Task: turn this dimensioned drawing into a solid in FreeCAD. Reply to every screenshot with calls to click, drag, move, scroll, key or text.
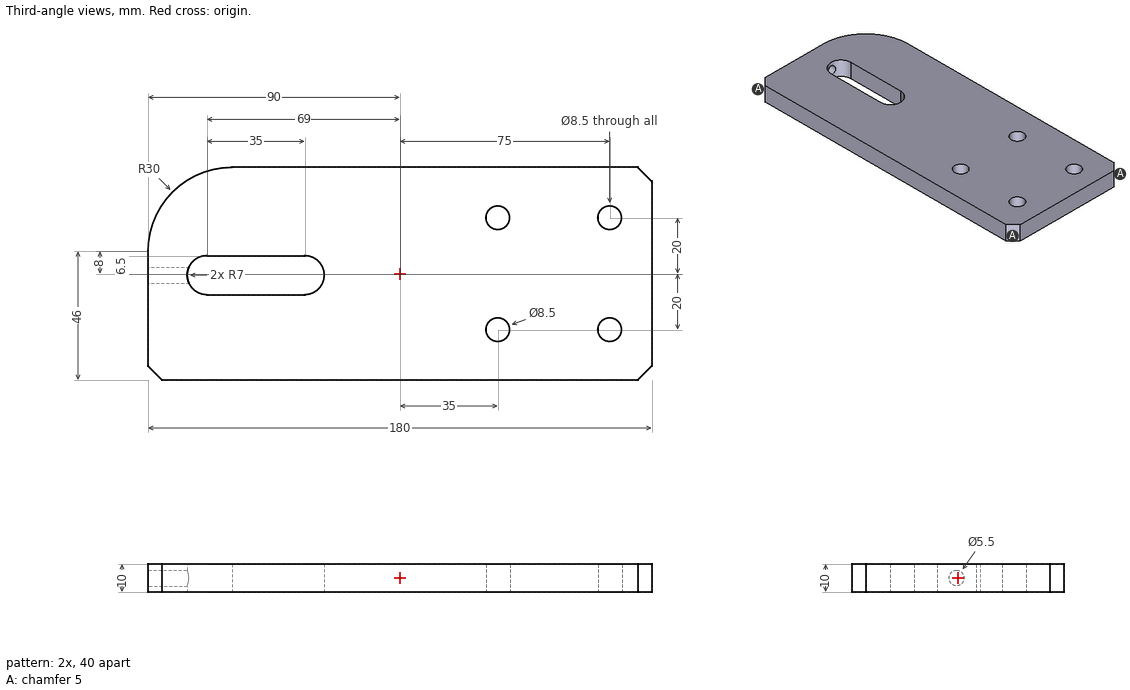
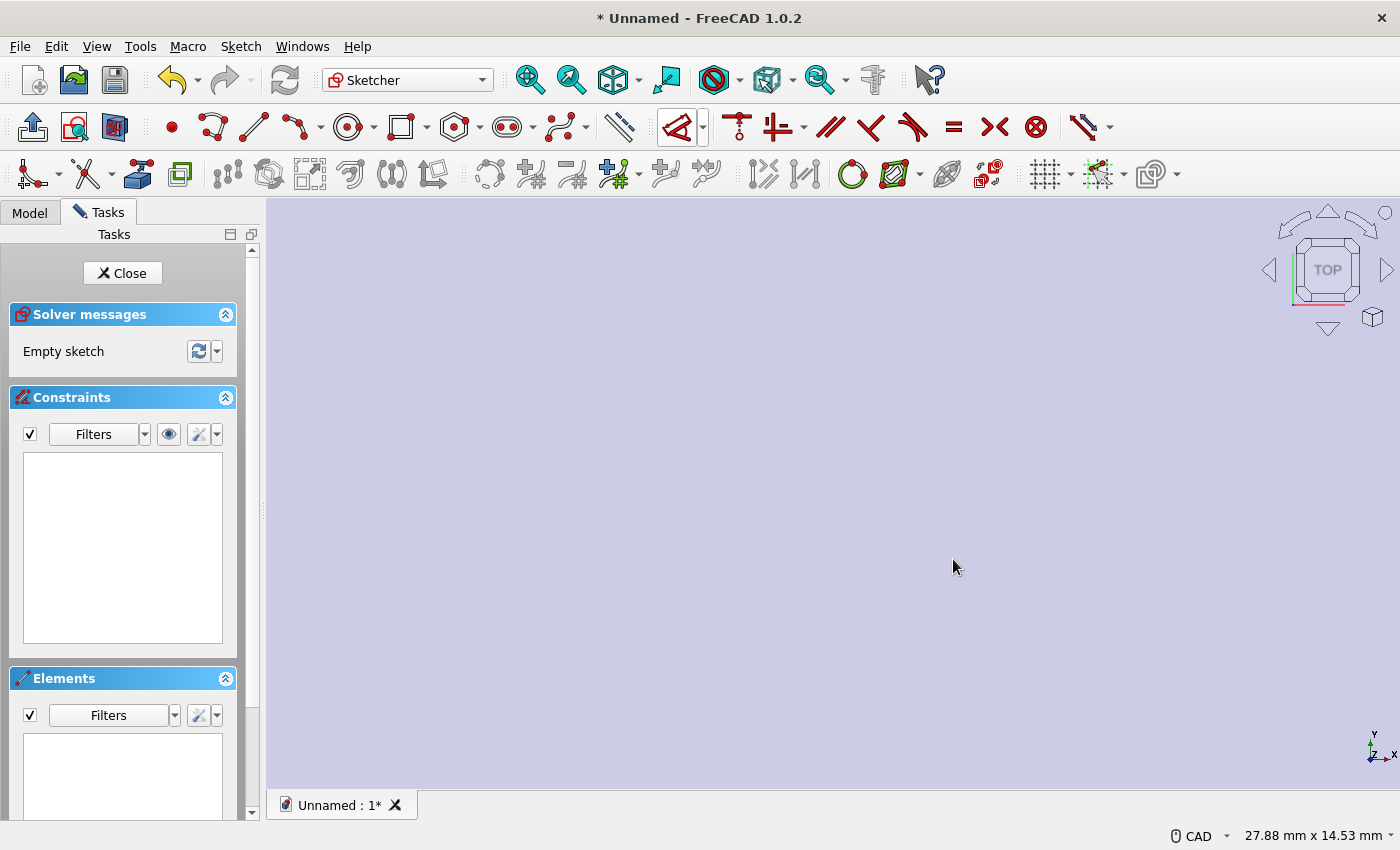
key(g)
key(c)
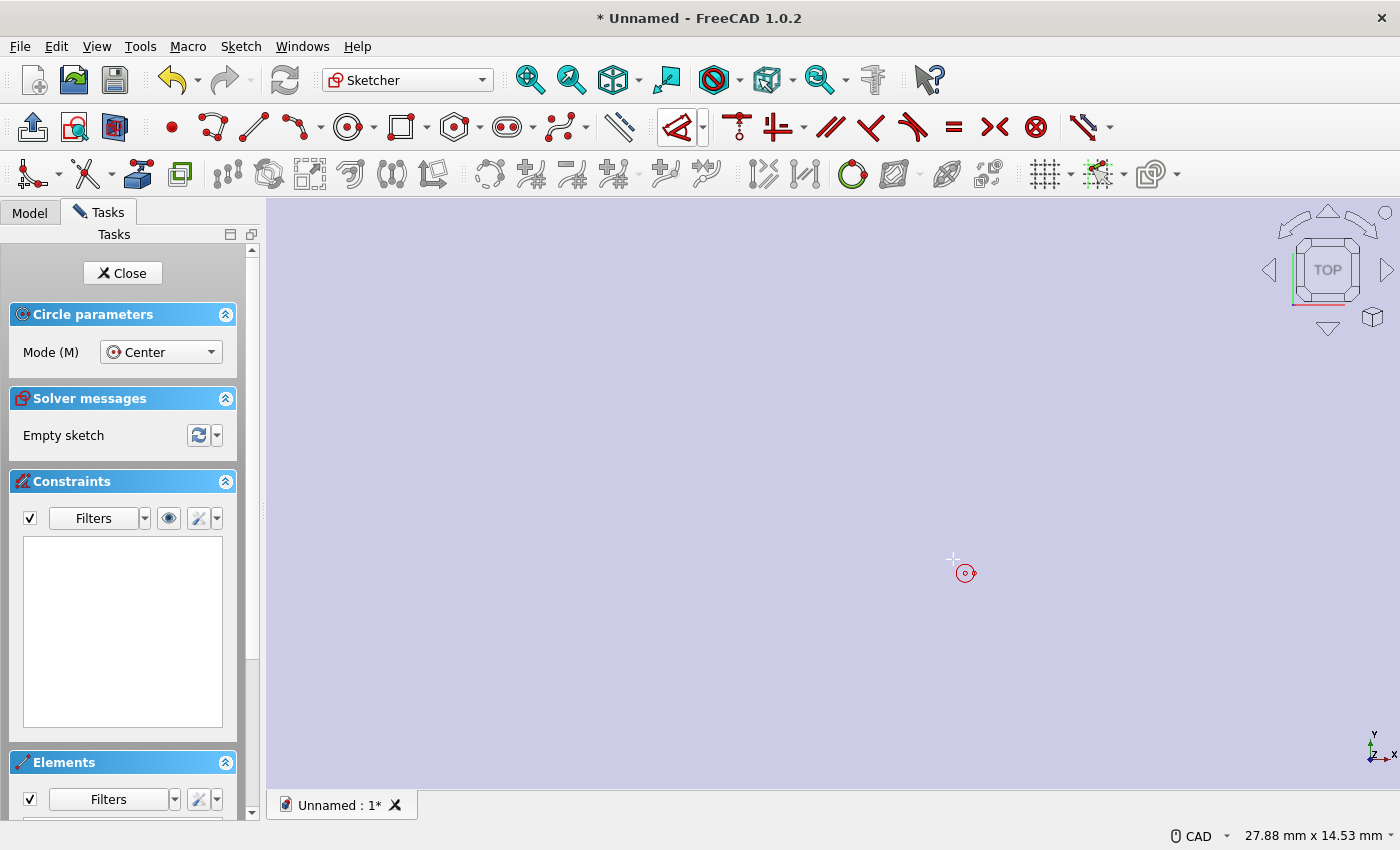
click(753, 483)
click(876, 361)
key(Escape)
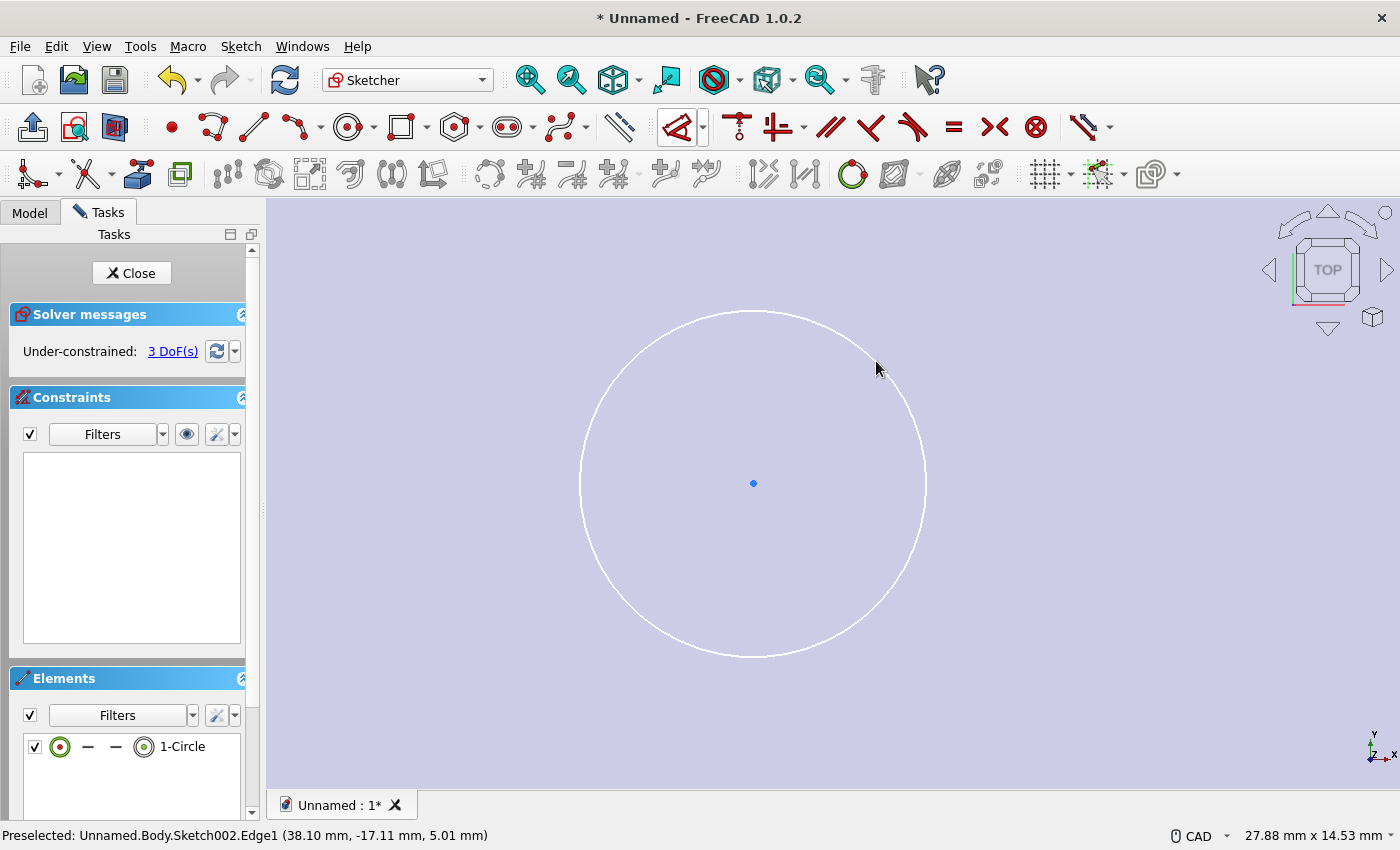
click(875, 361)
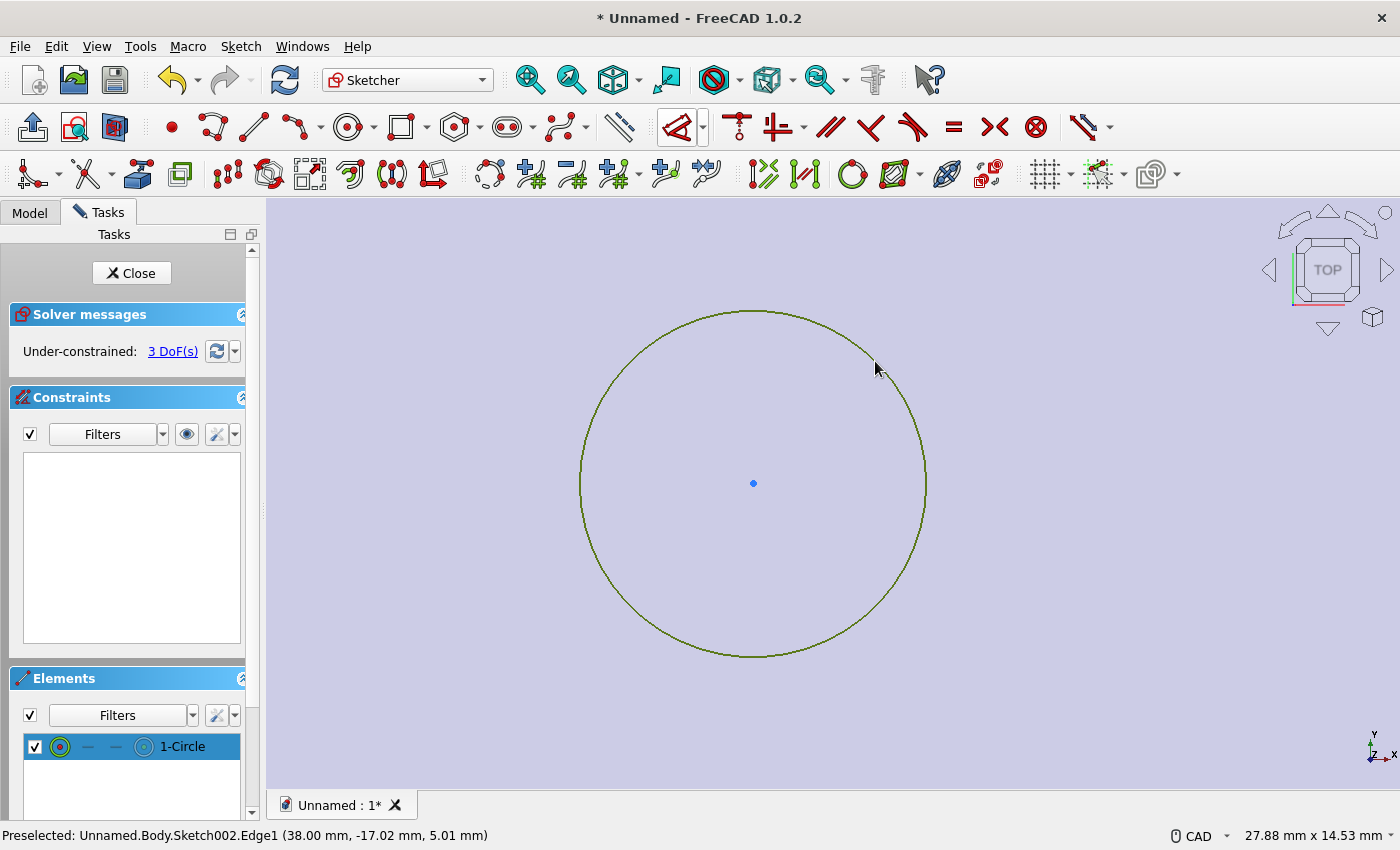
click(702, 128)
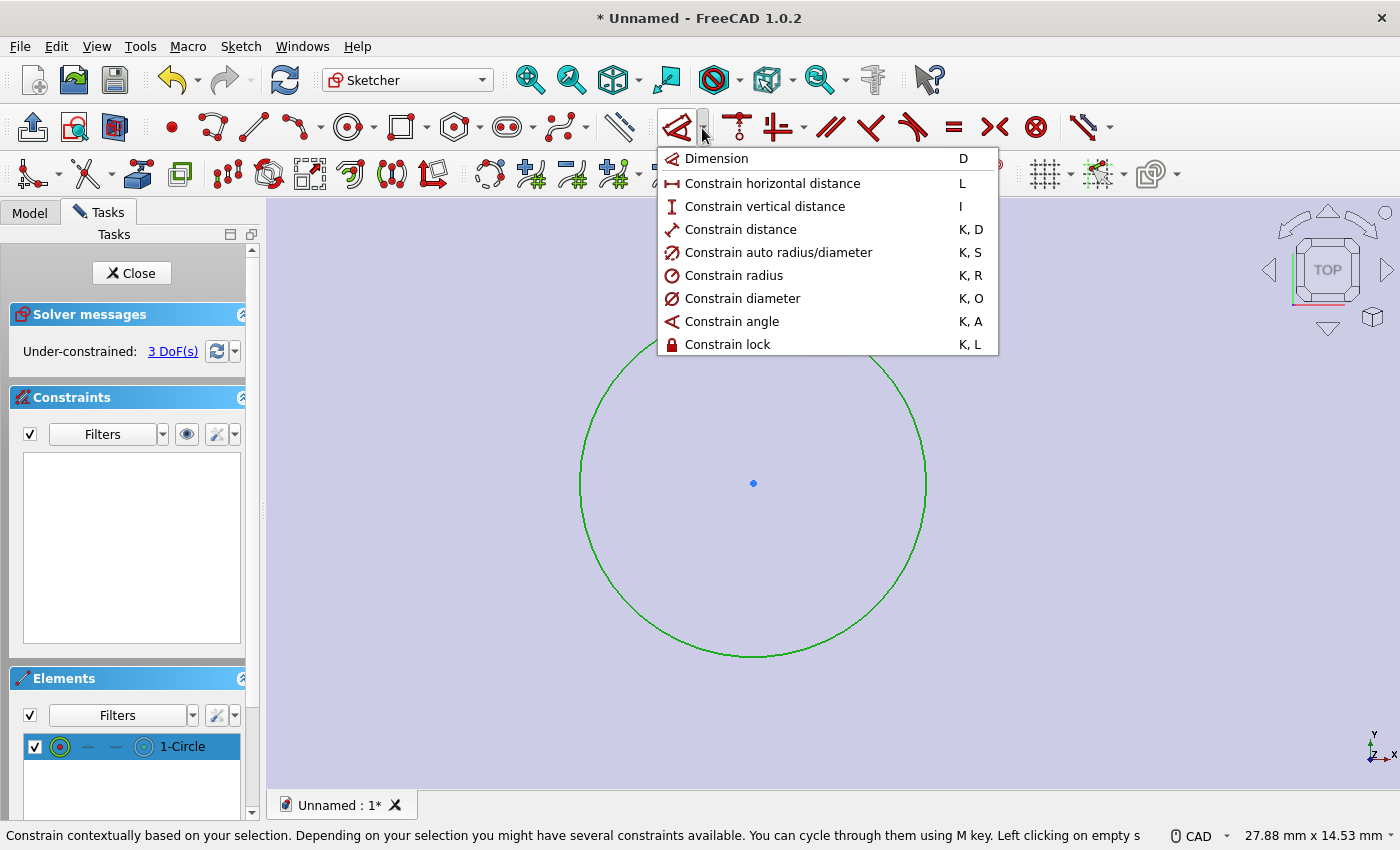
click(828, 298)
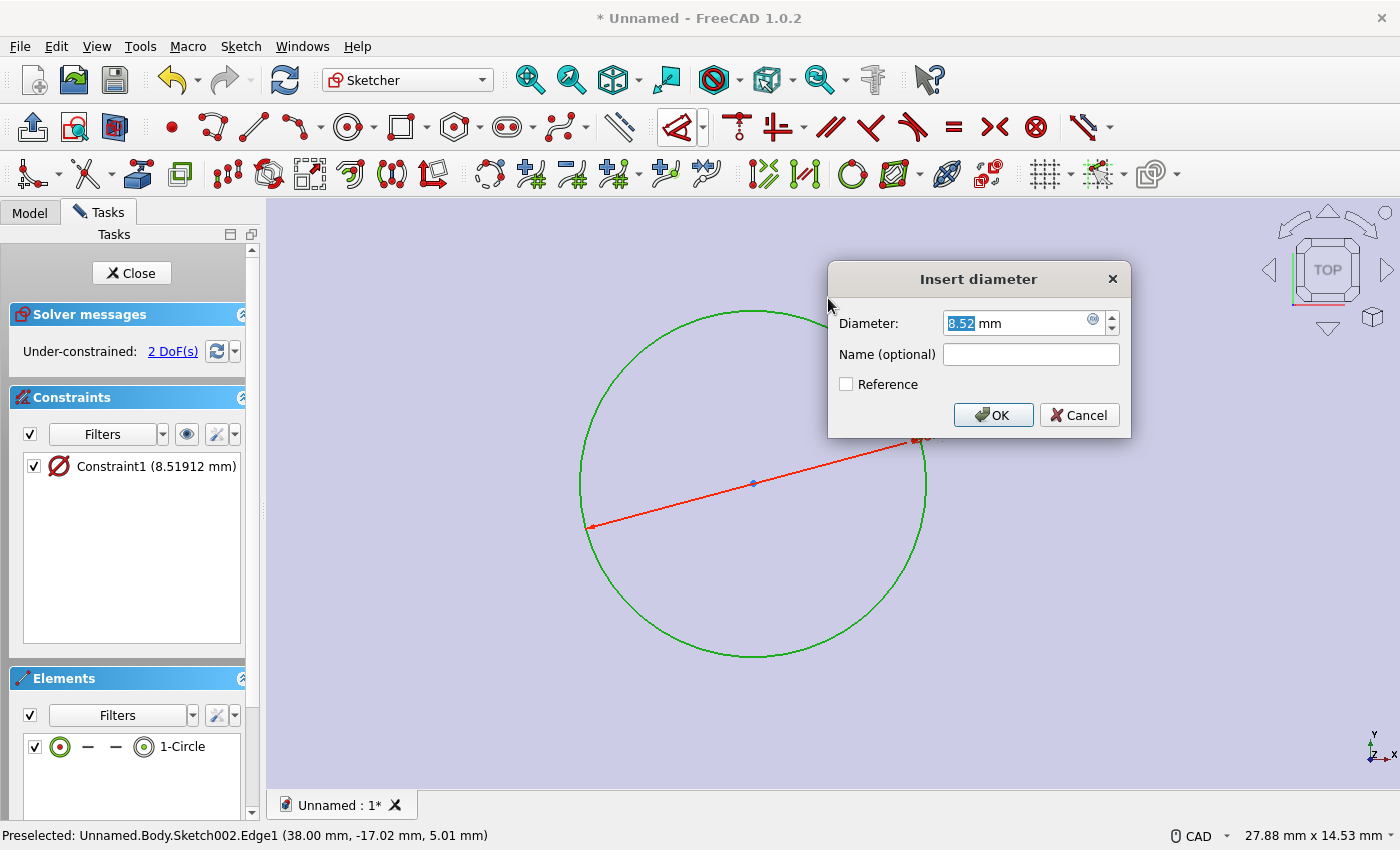
text(8.5)
key(Return)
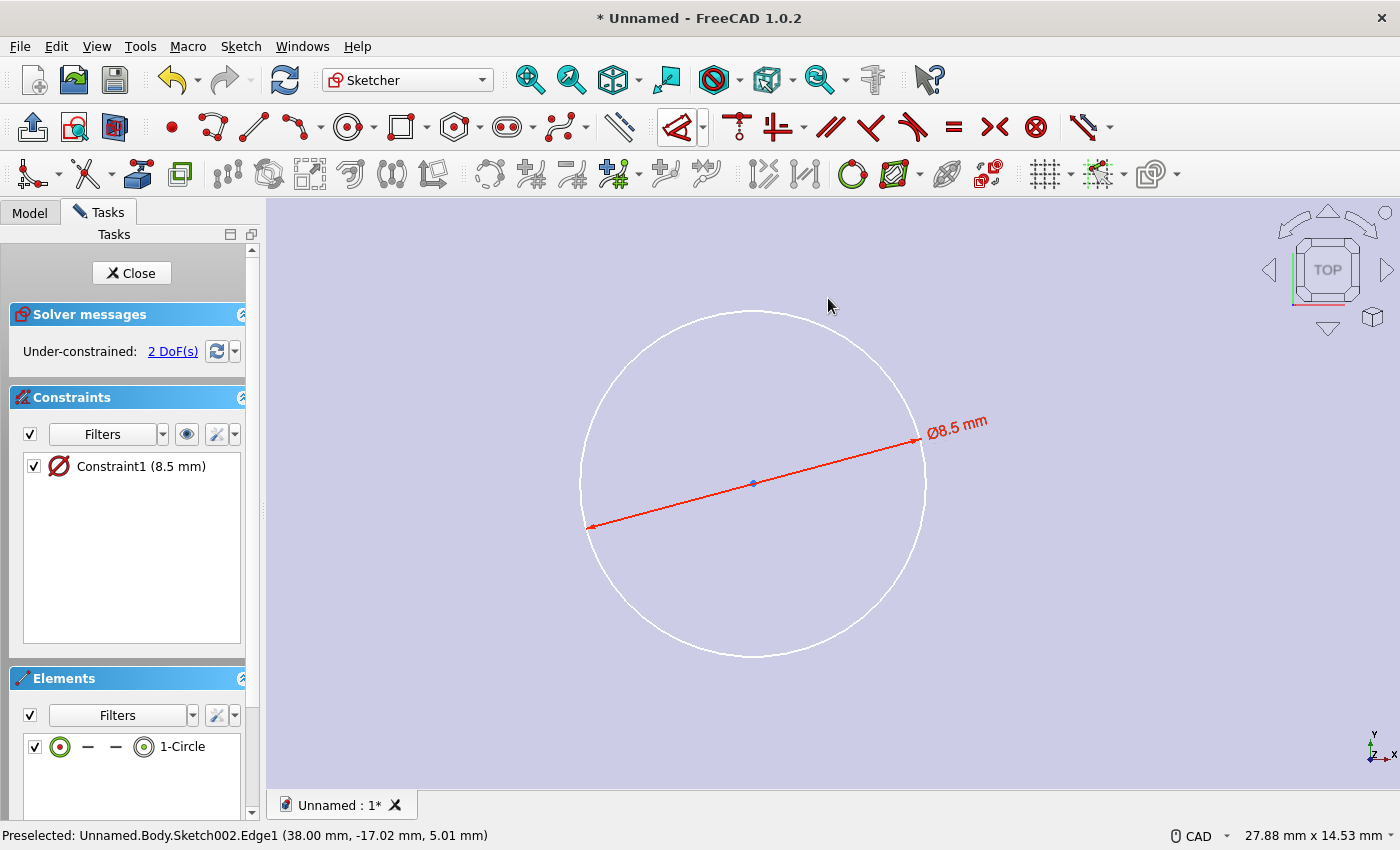
click(753, 484)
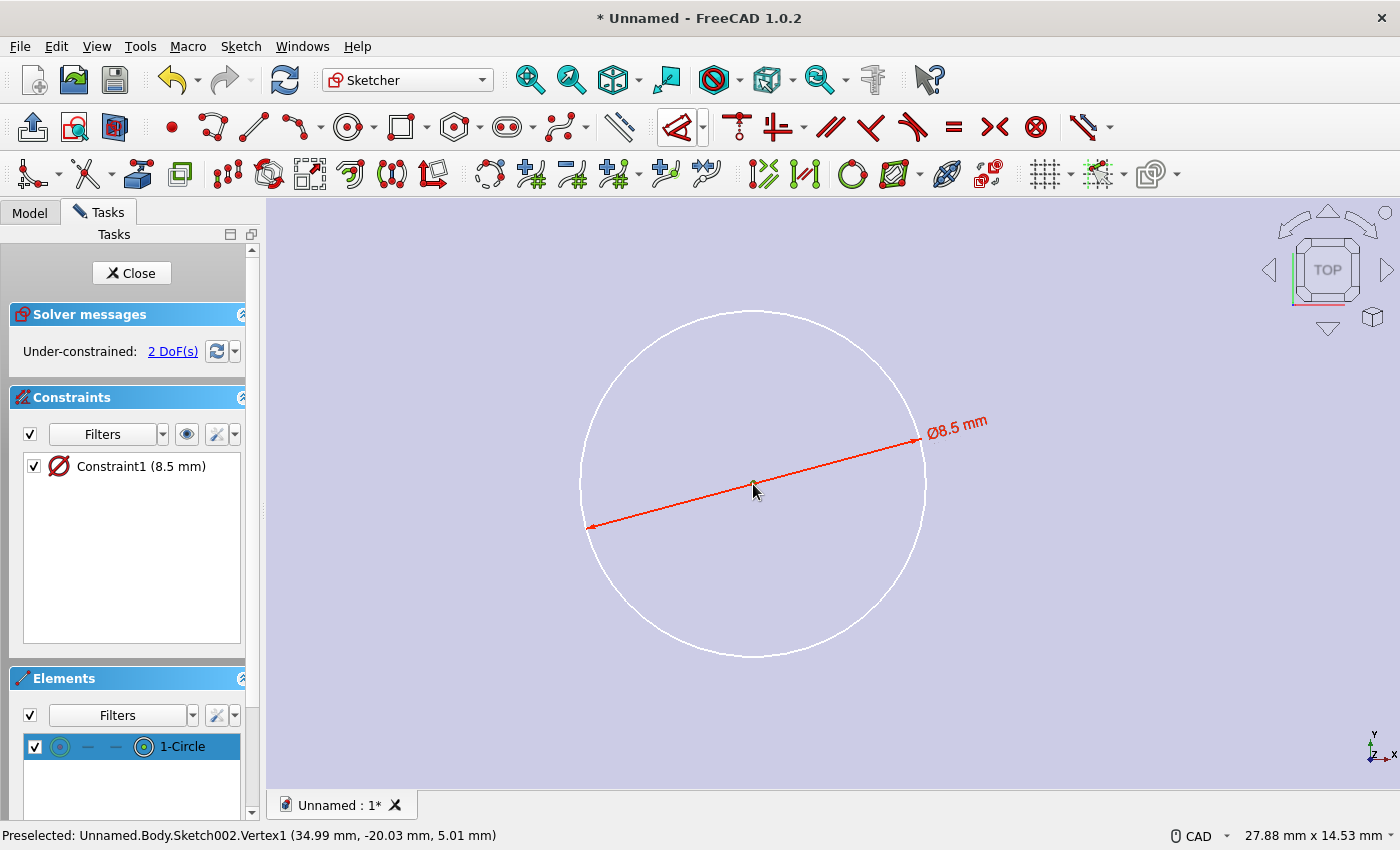
key(l)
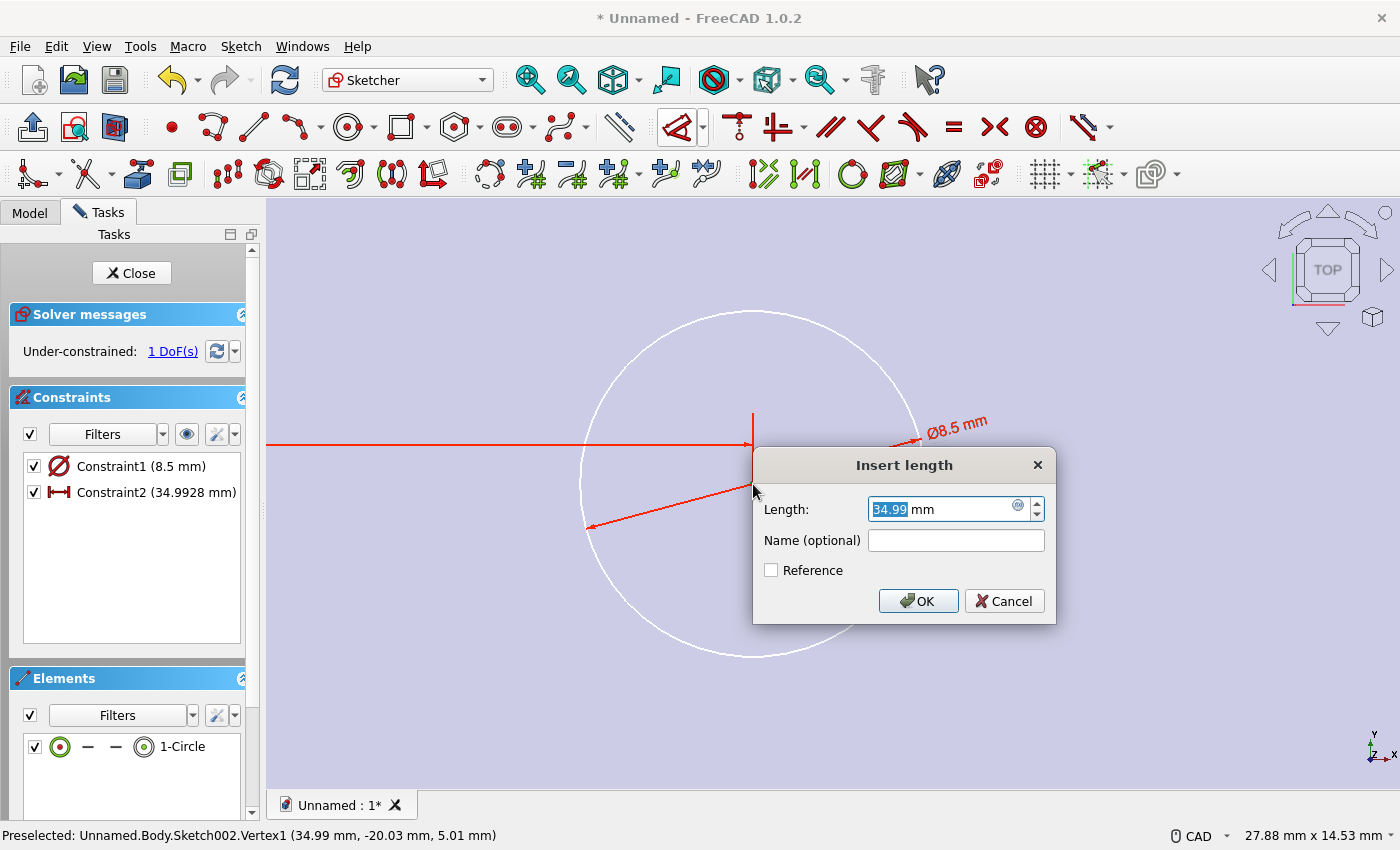
text(35)
key(Return)